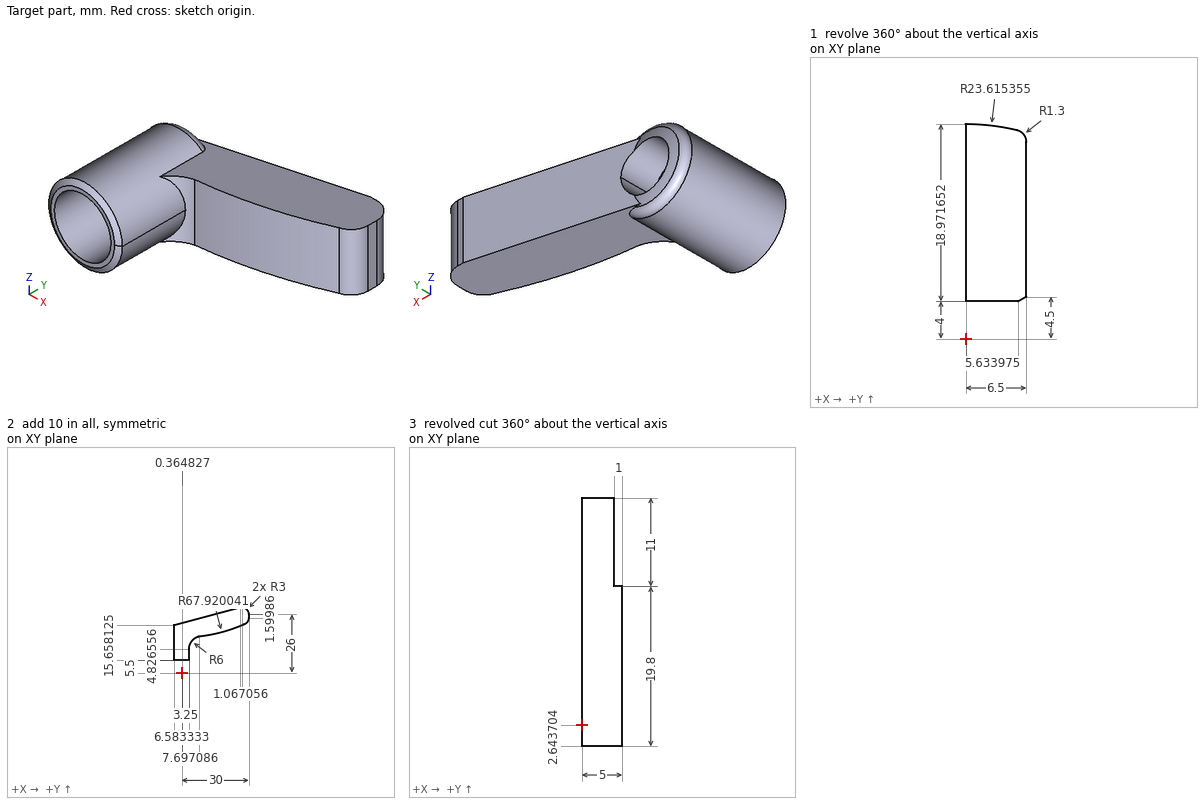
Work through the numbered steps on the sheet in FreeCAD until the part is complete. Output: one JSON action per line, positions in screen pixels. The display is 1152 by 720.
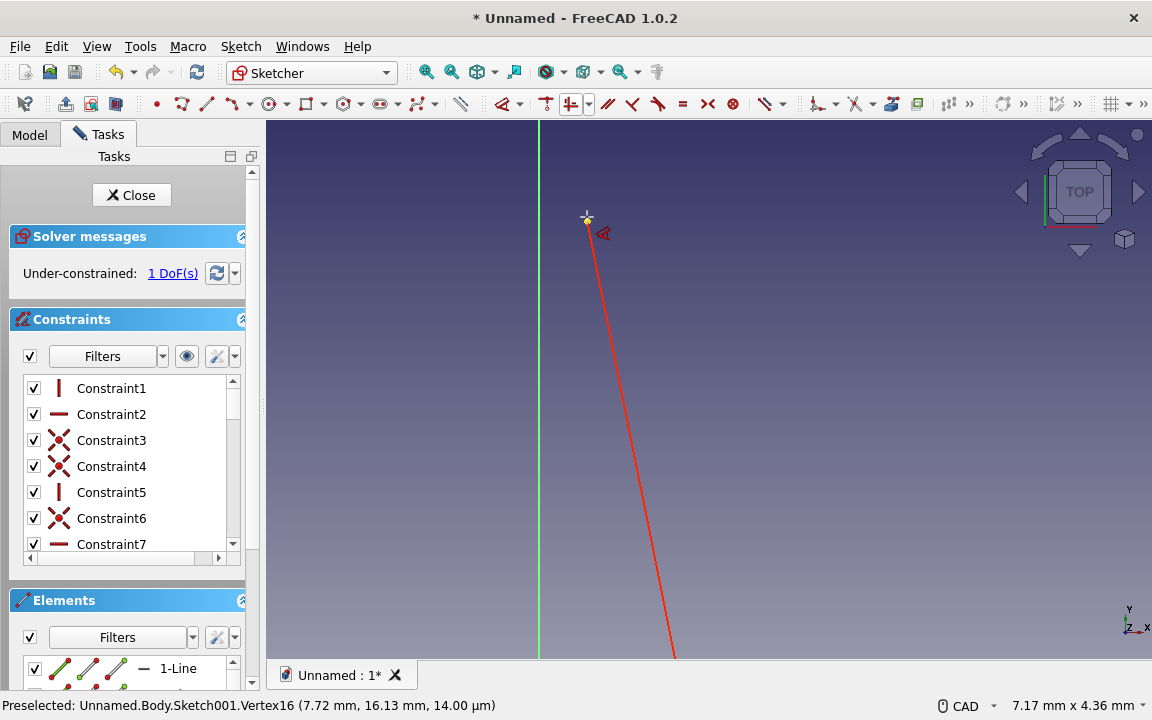
{"action": "left_click", "coordinate": [587, 222]}
{"action": "left_click", "coordinate": [563, 188]}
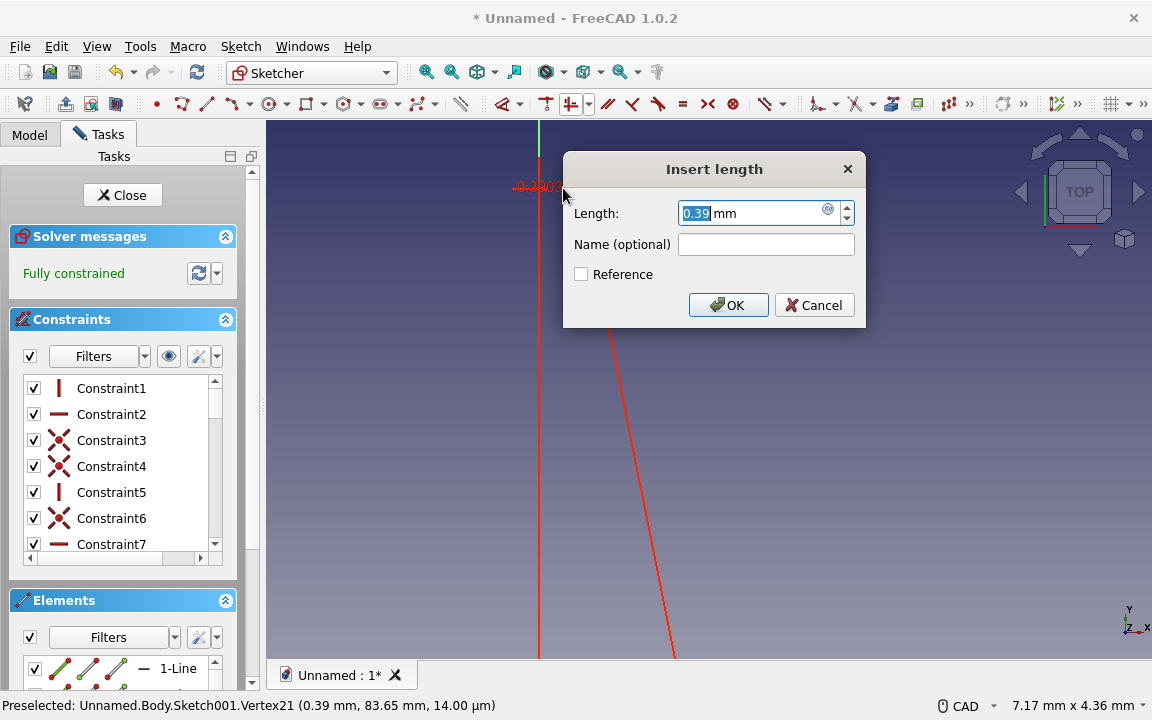
{"action": "type", "text": "0.364827"}
{"action": "key", "text": "Return"}
{"action": "key", "text": "Escape"}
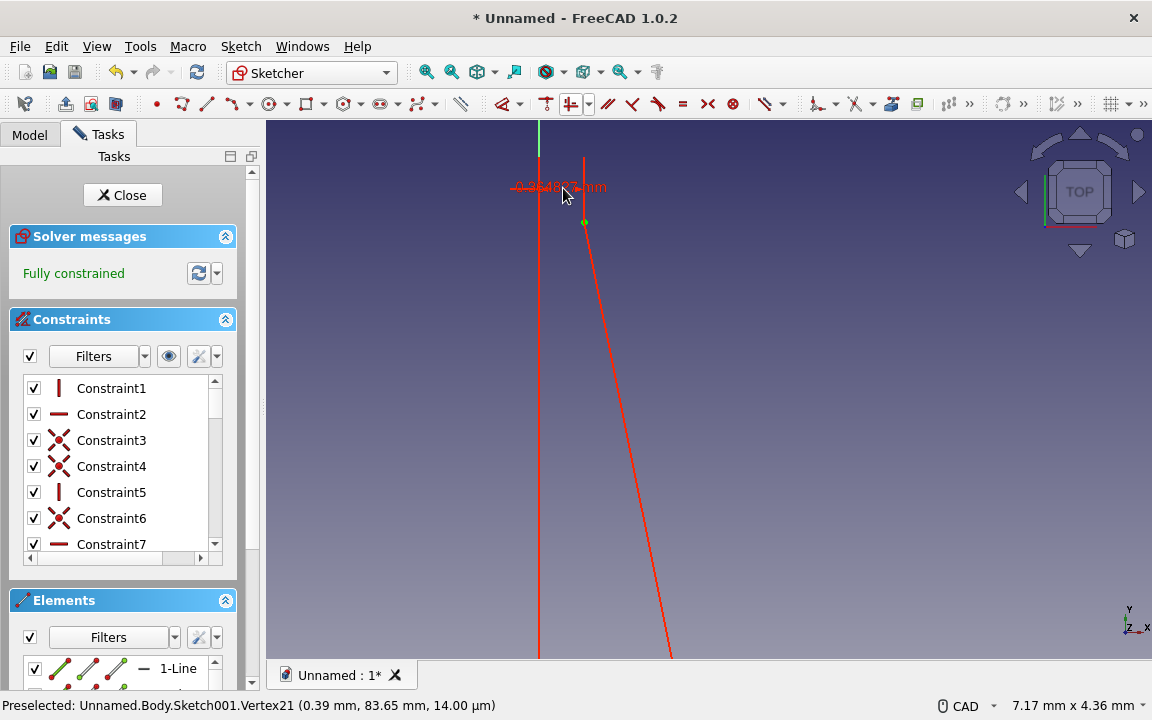
{"action": "left_click", "coordinate": [123, 195]}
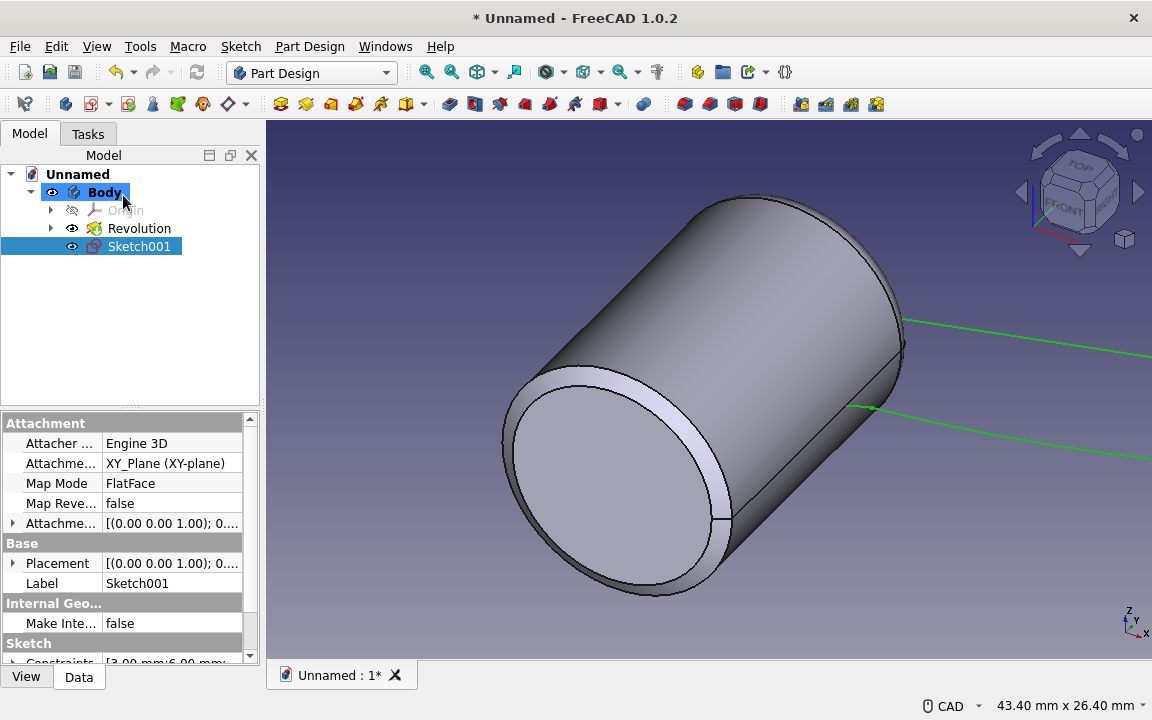
{"action": "left_click", "coordinate": [281, 104]}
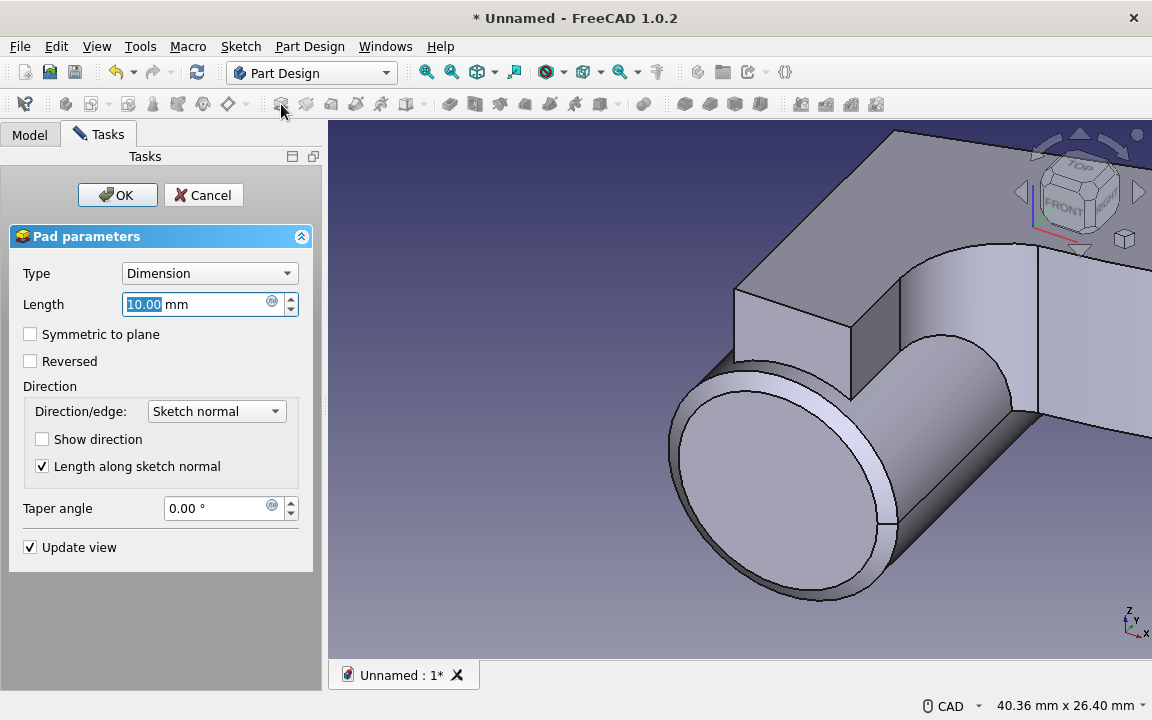
{"action": "type", "text": "10"}
{"action": "key", "text": "Tab"}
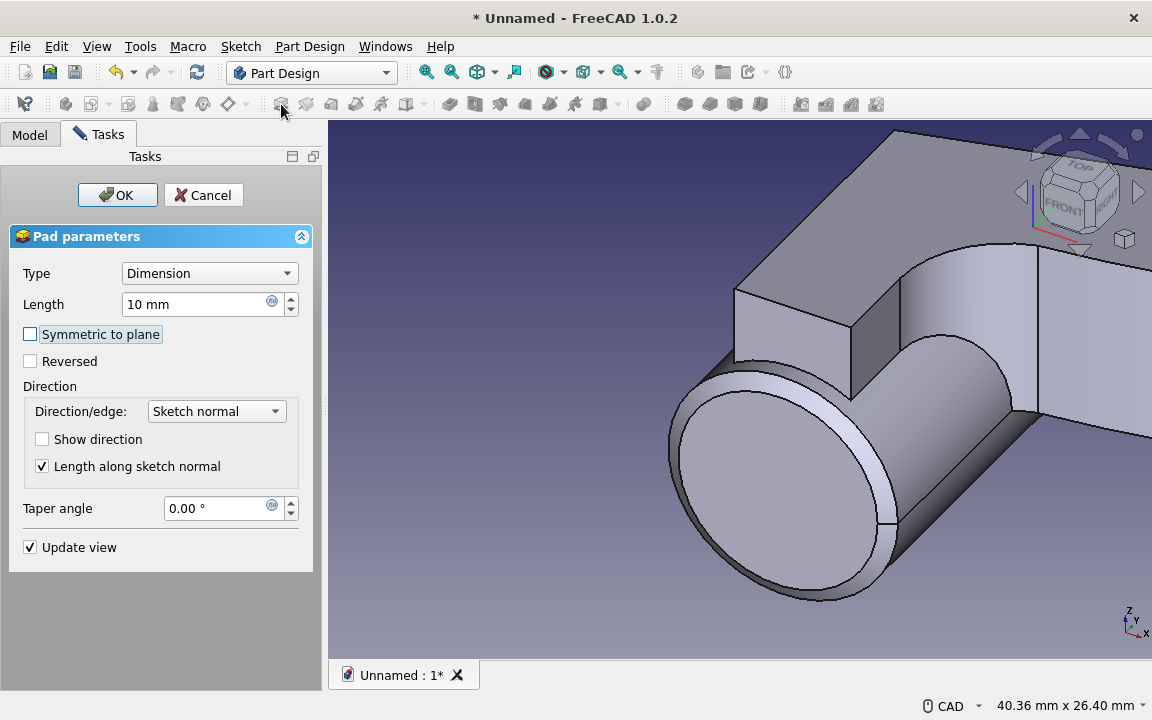
{"action": "left_click", "coordinate": [31, 334]}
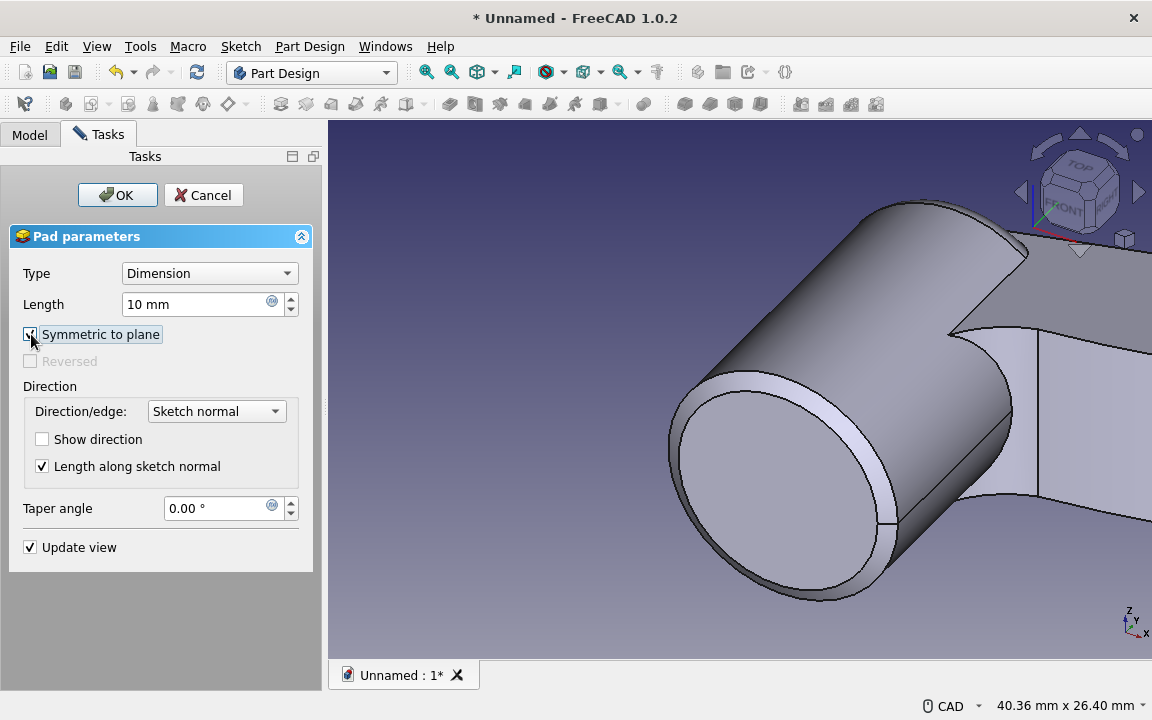
{"action": "left_click", "coordinate": [118, 195]}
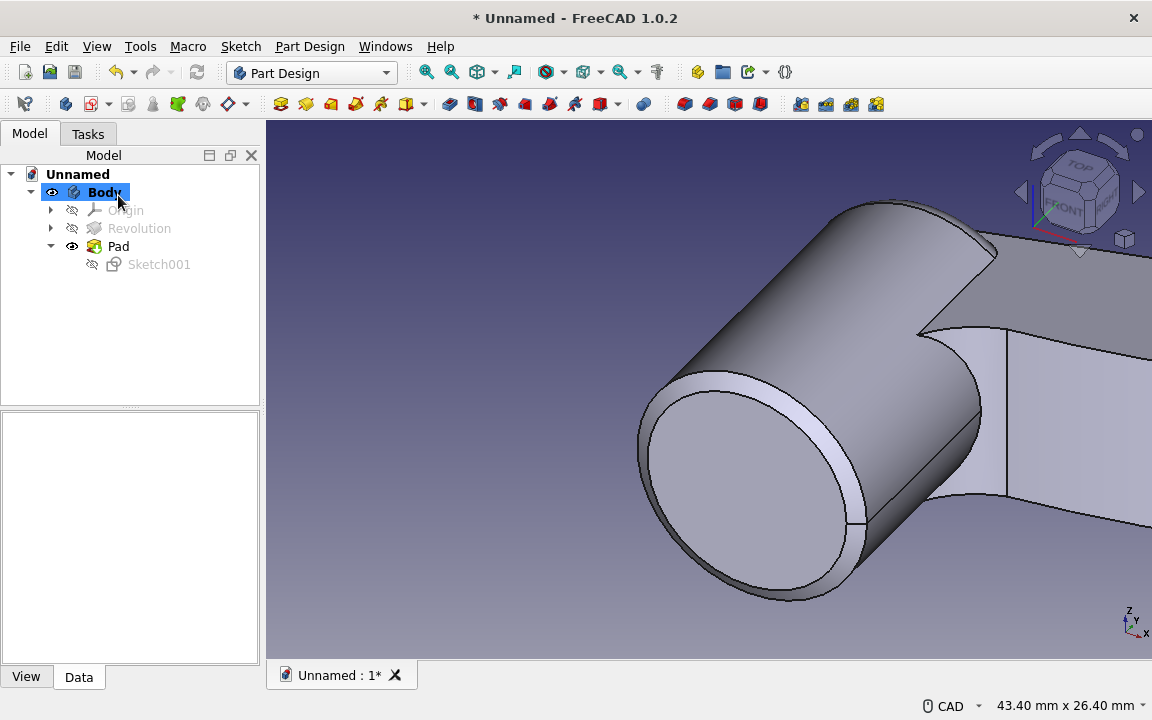
{"action": "key", "text": "v f"}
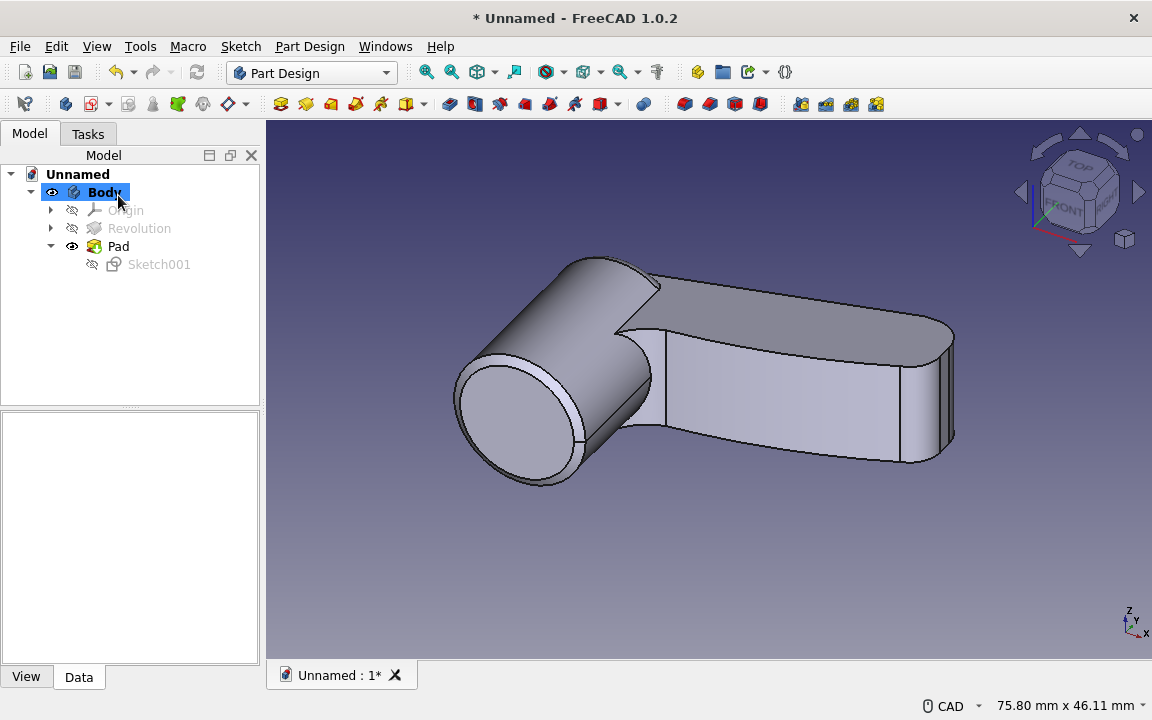
{"action": "left_click", "coordinate": [90, 104]}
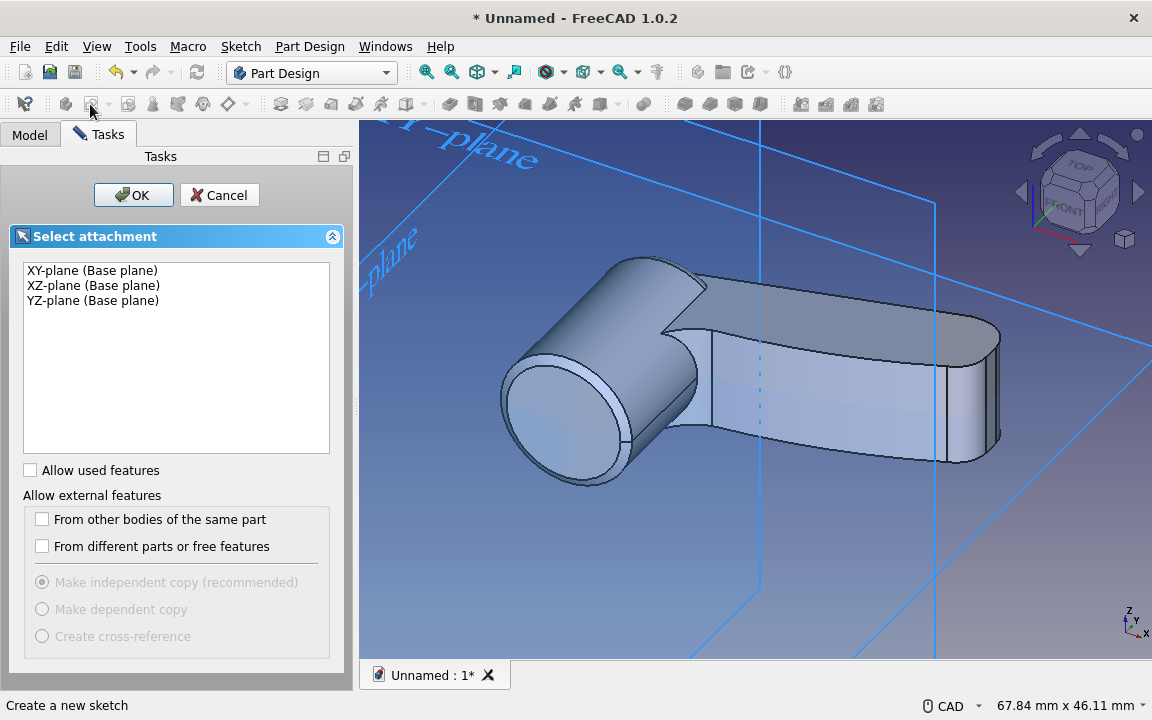
{"action": "left_click", "coordinate": [84, 270]}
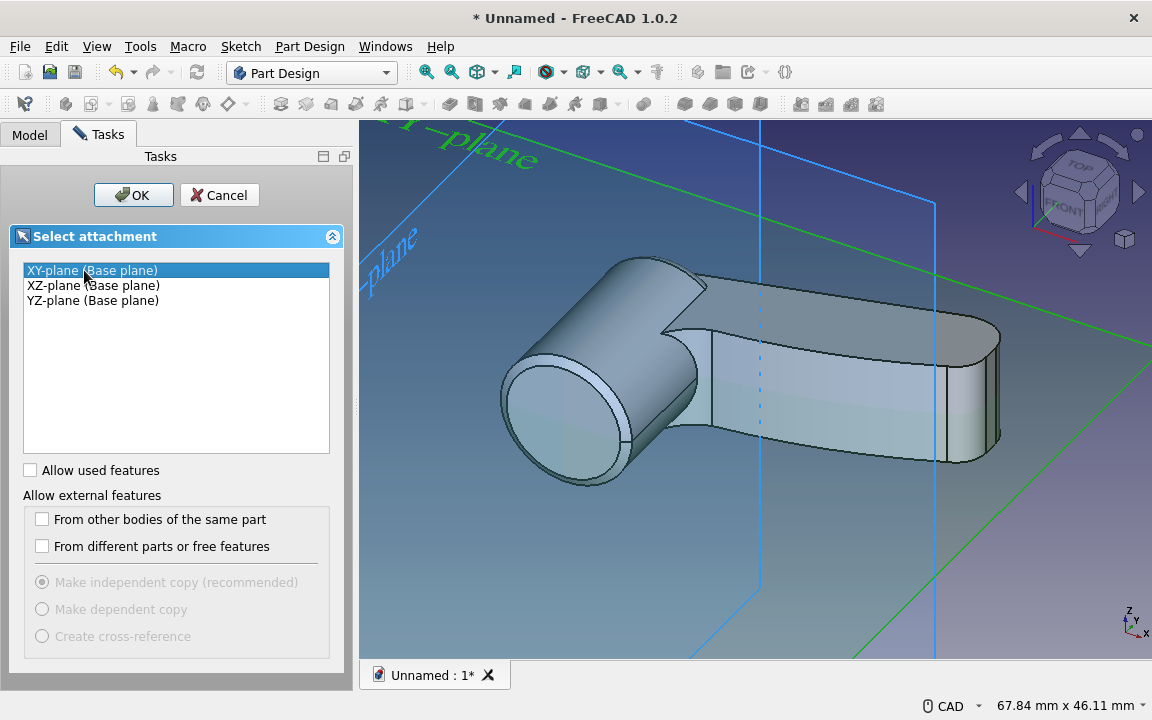
{"action": "left_click", "coordinate": [134, 195]}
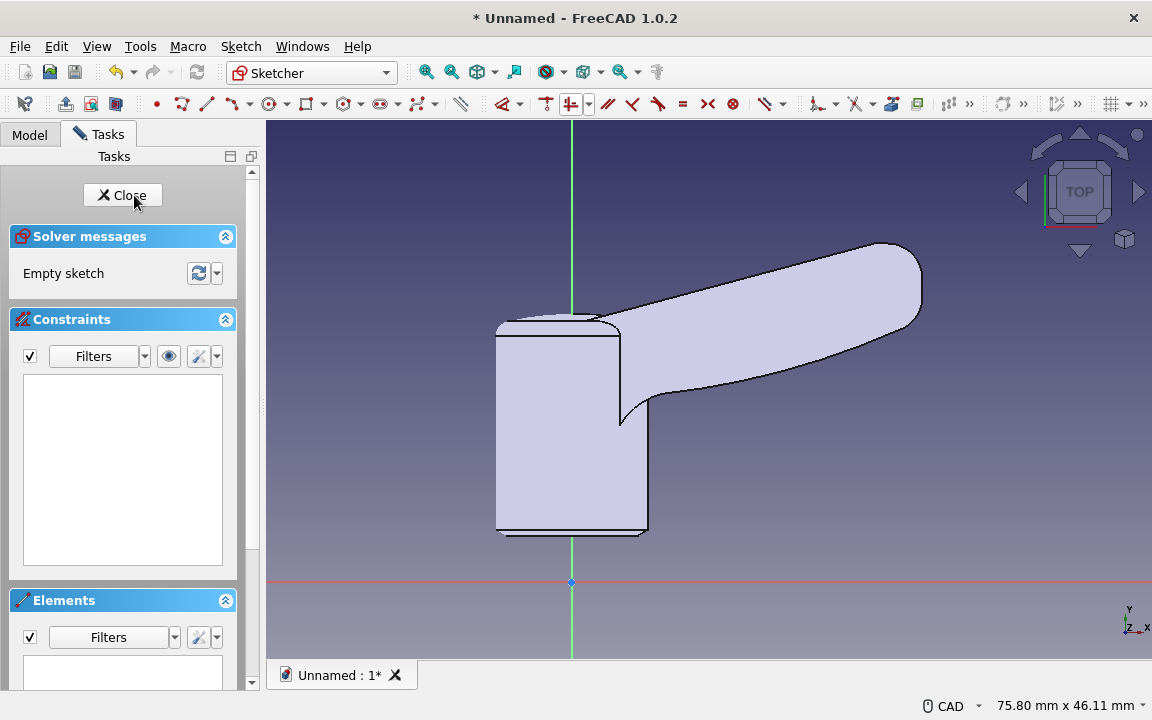
{"action": "key", "text": "q s"}